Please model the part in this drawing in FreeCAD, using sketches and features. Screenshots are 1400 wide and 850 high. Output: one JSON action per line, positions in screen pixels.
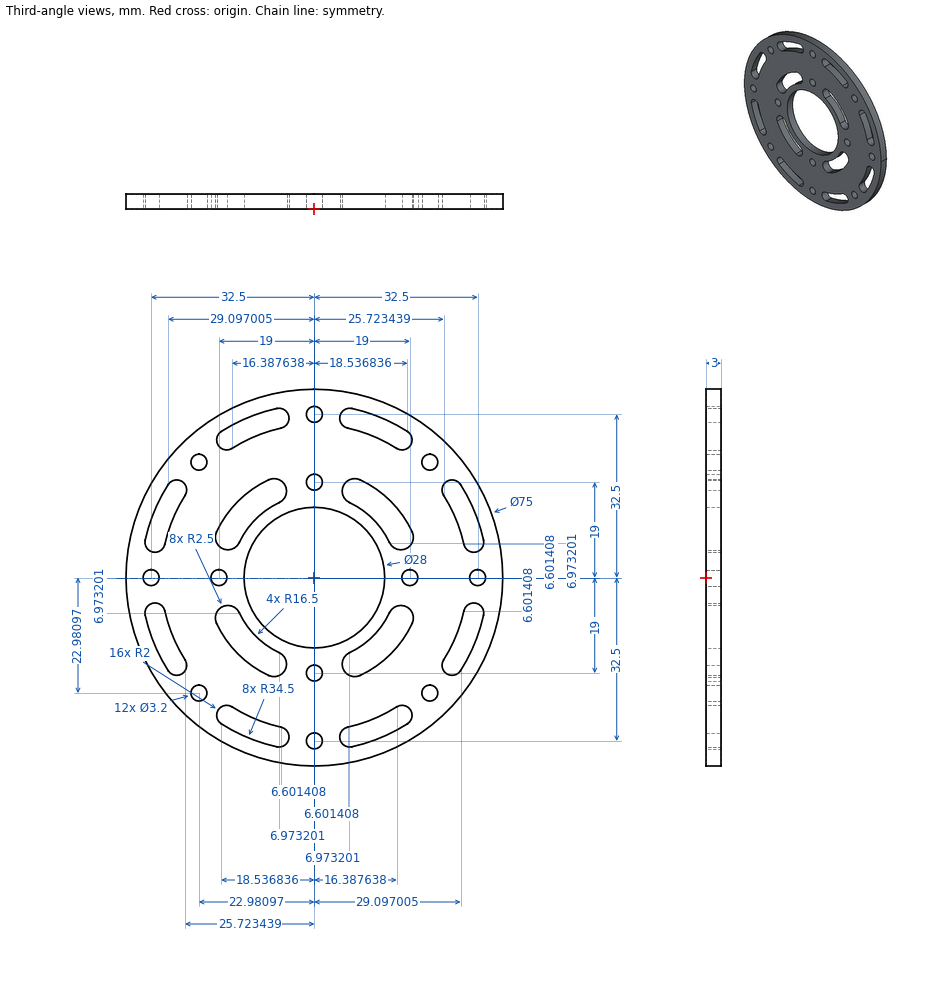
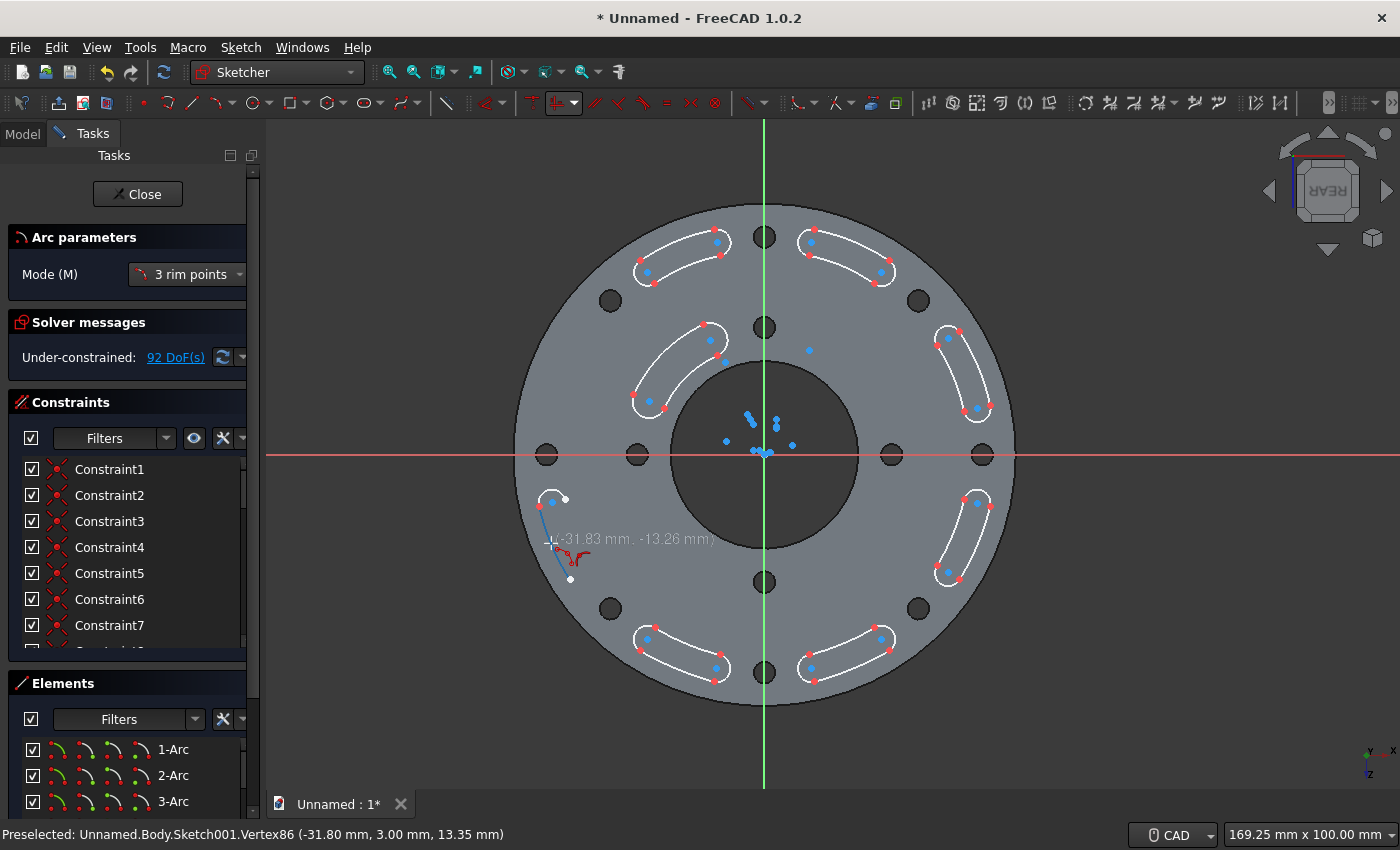
{"action": "left_click", "coordinate": [570, 580]}
{"action": "left_click", "coordinate": [592, 565]}
{"action": "left_click", "coordinate": [588, 583]}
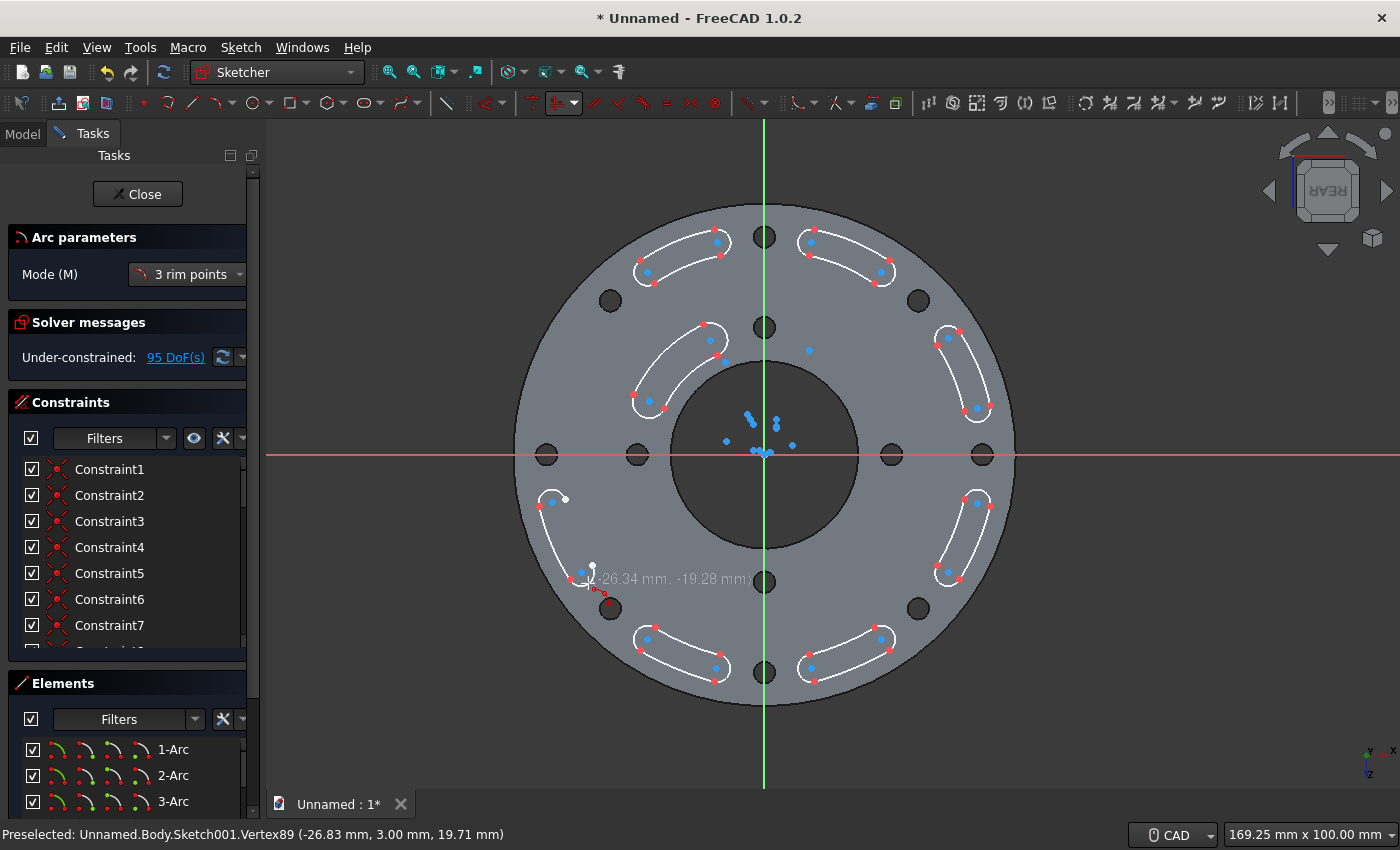
{"action": "left_click", "coordinate": [592, 566]}
{"action": "left_click", "coordinate": [565, 500]}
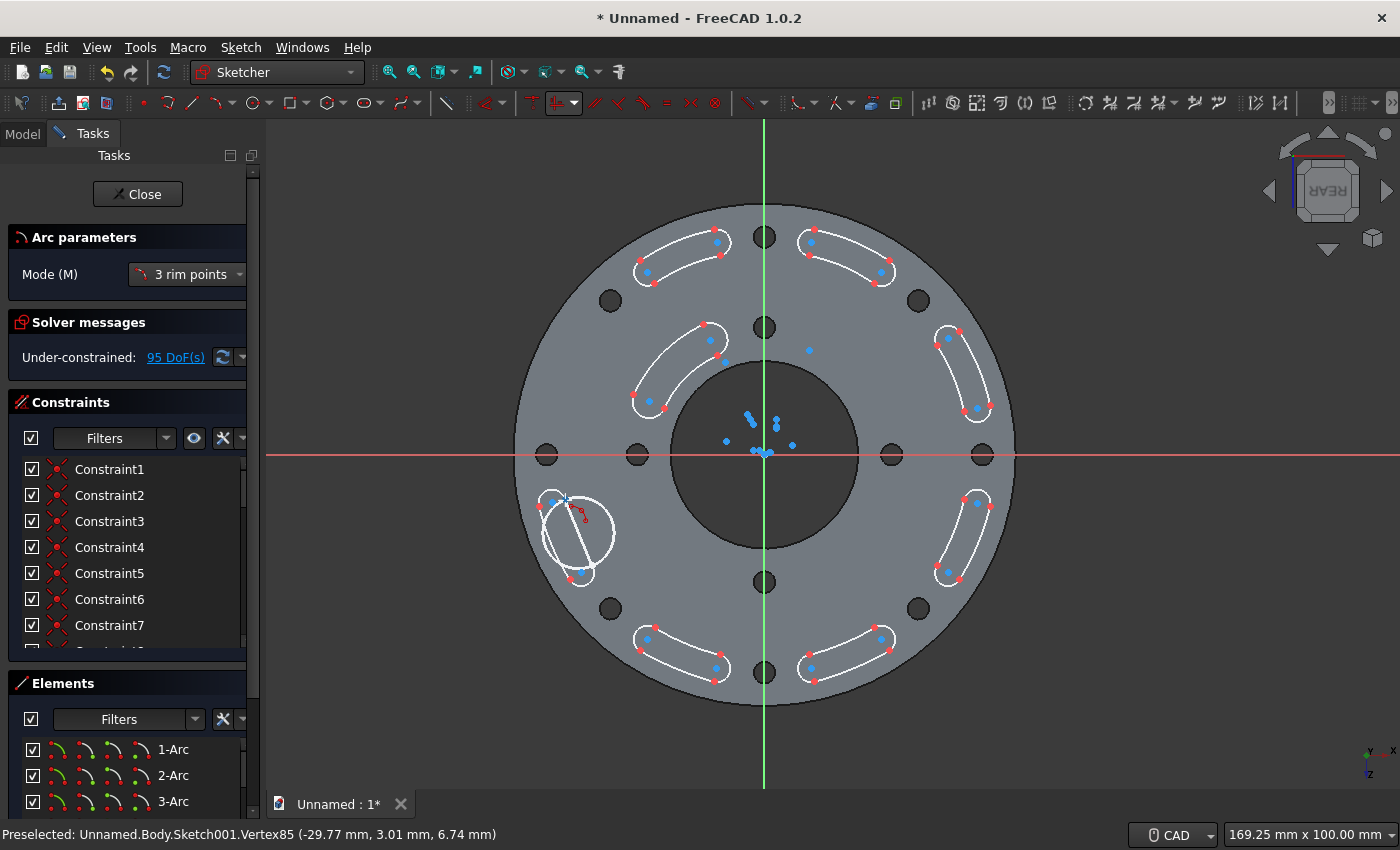
{"action": "scroll", "coordinate": [576, 533], "scroll_direction": "up", "scroll_amount": 9}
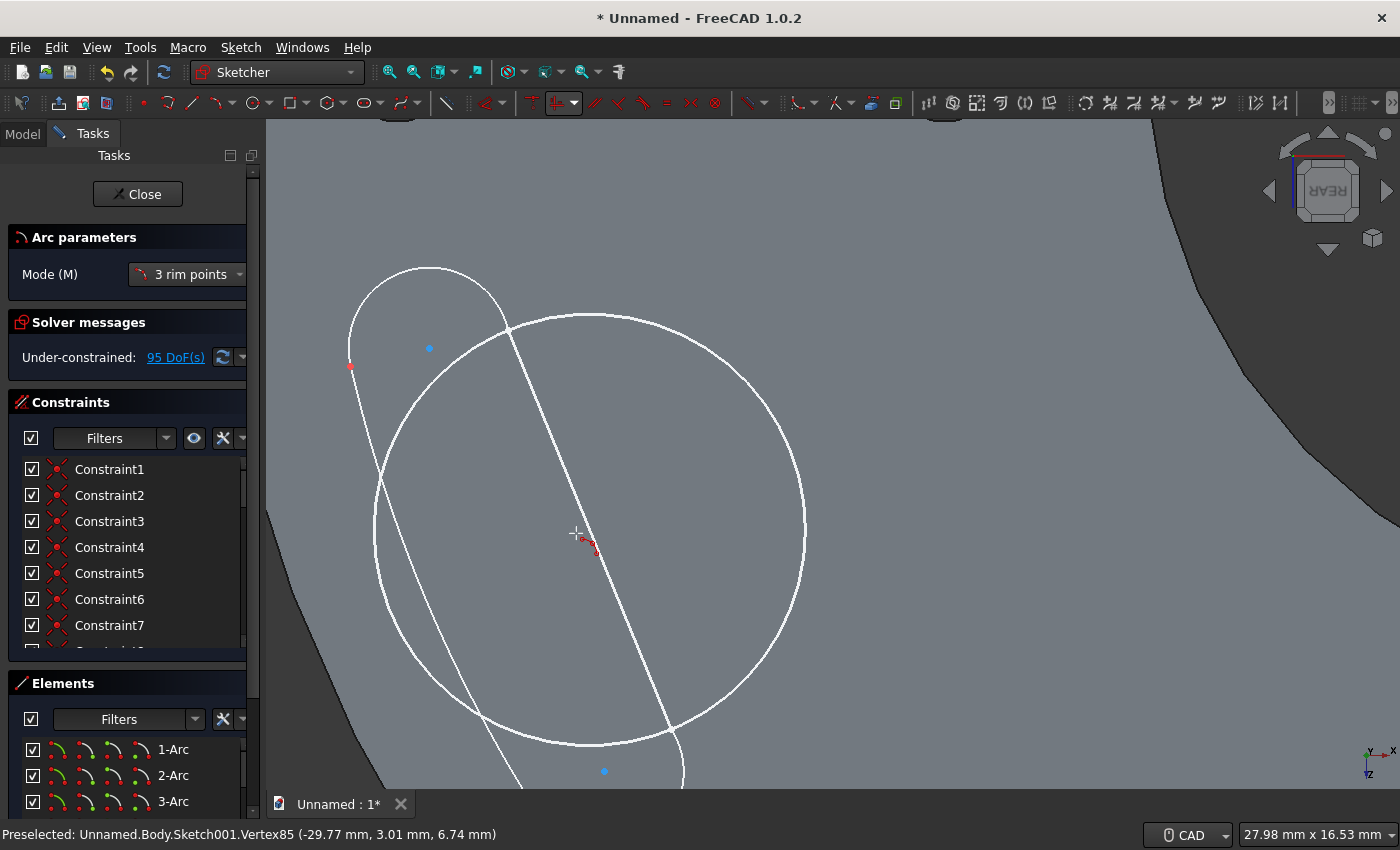
{"action": "left_click", "coordinate": [573, 530]}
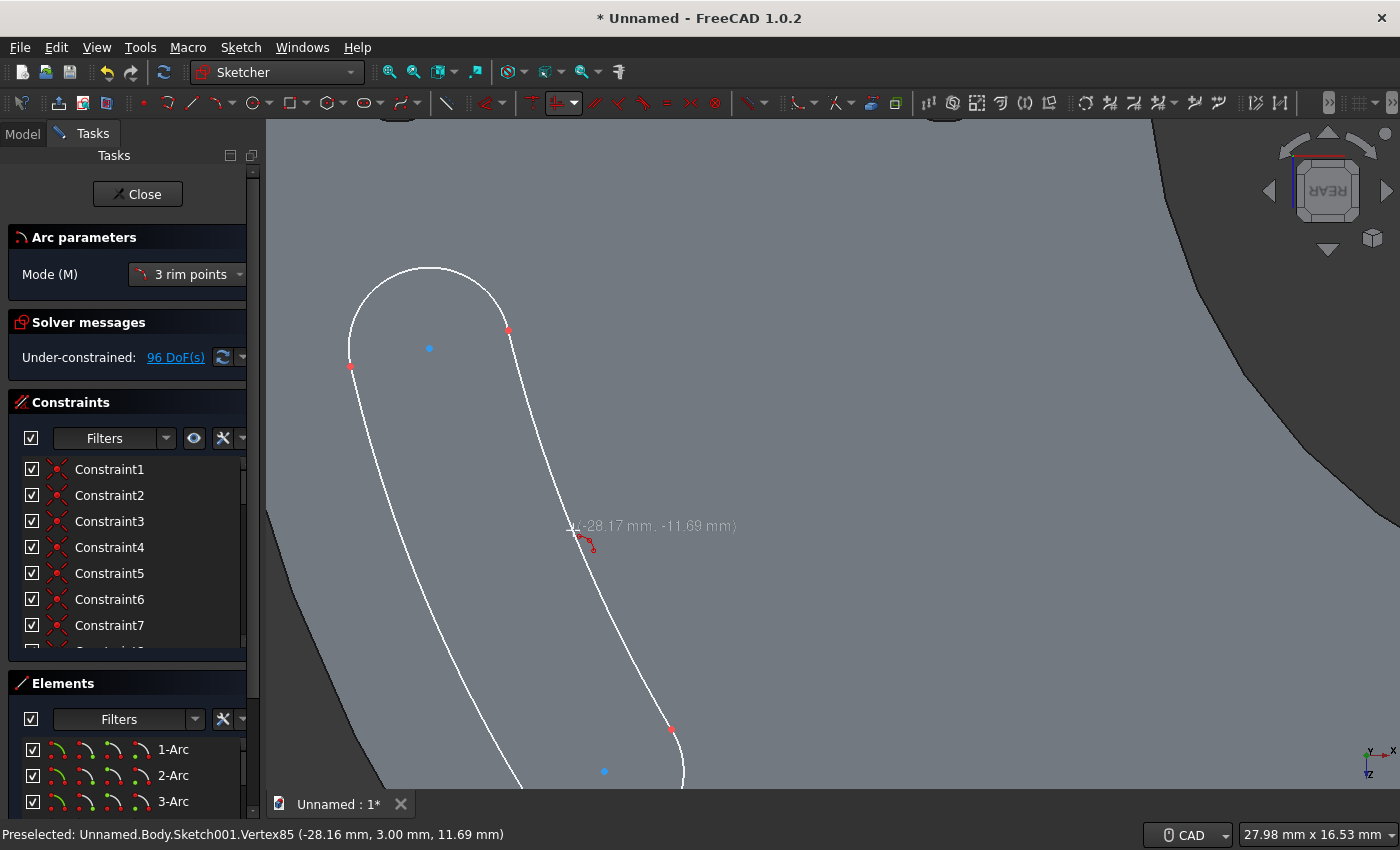
{"action": "scroll", "coordinate": [576, 533], "scroll_direction": "down", "scroll_amount": 9}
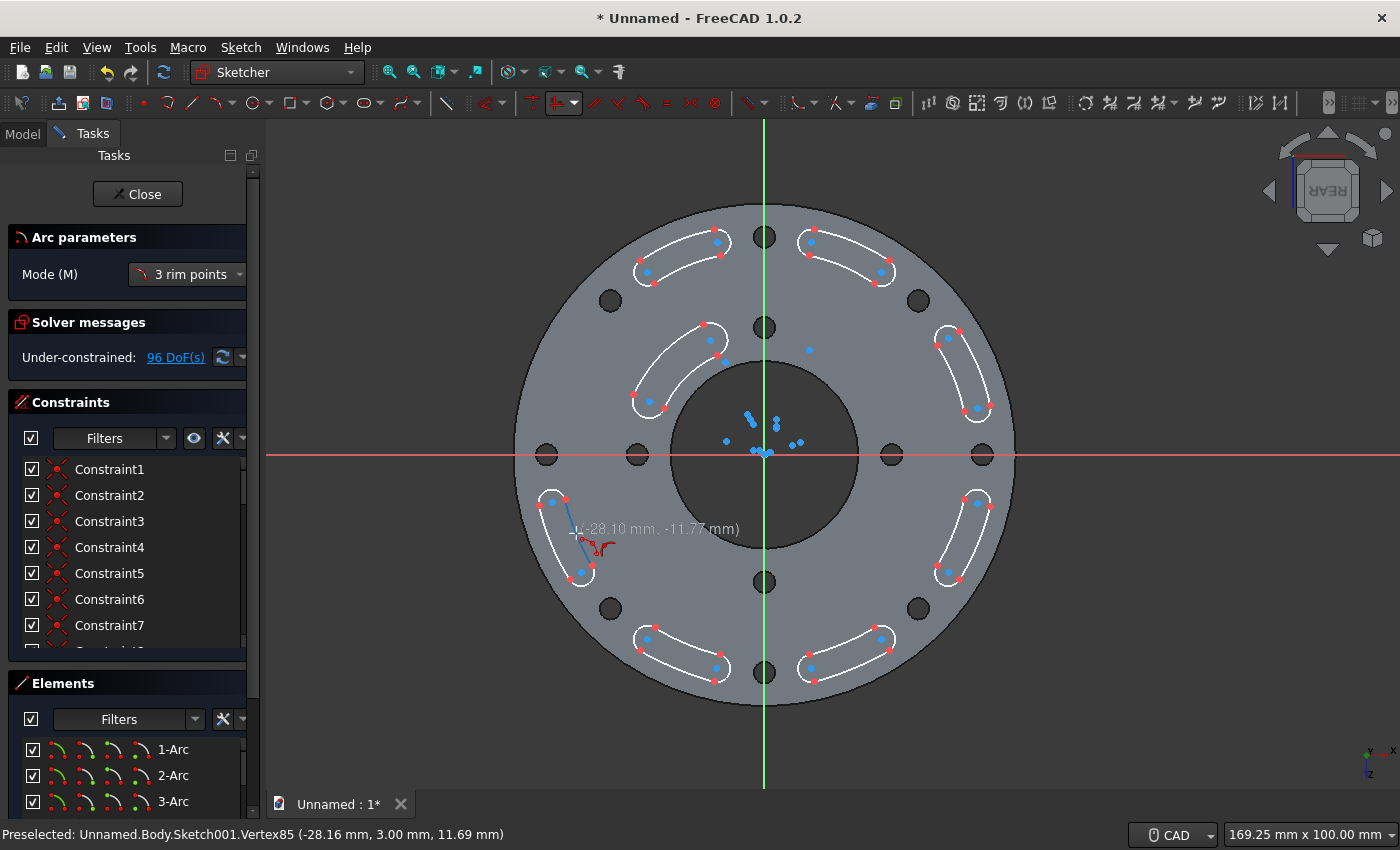
{"action": "left_click", "coordinate": [565, 411]}
{"action": "left_click", "coordinate": [592, 345]}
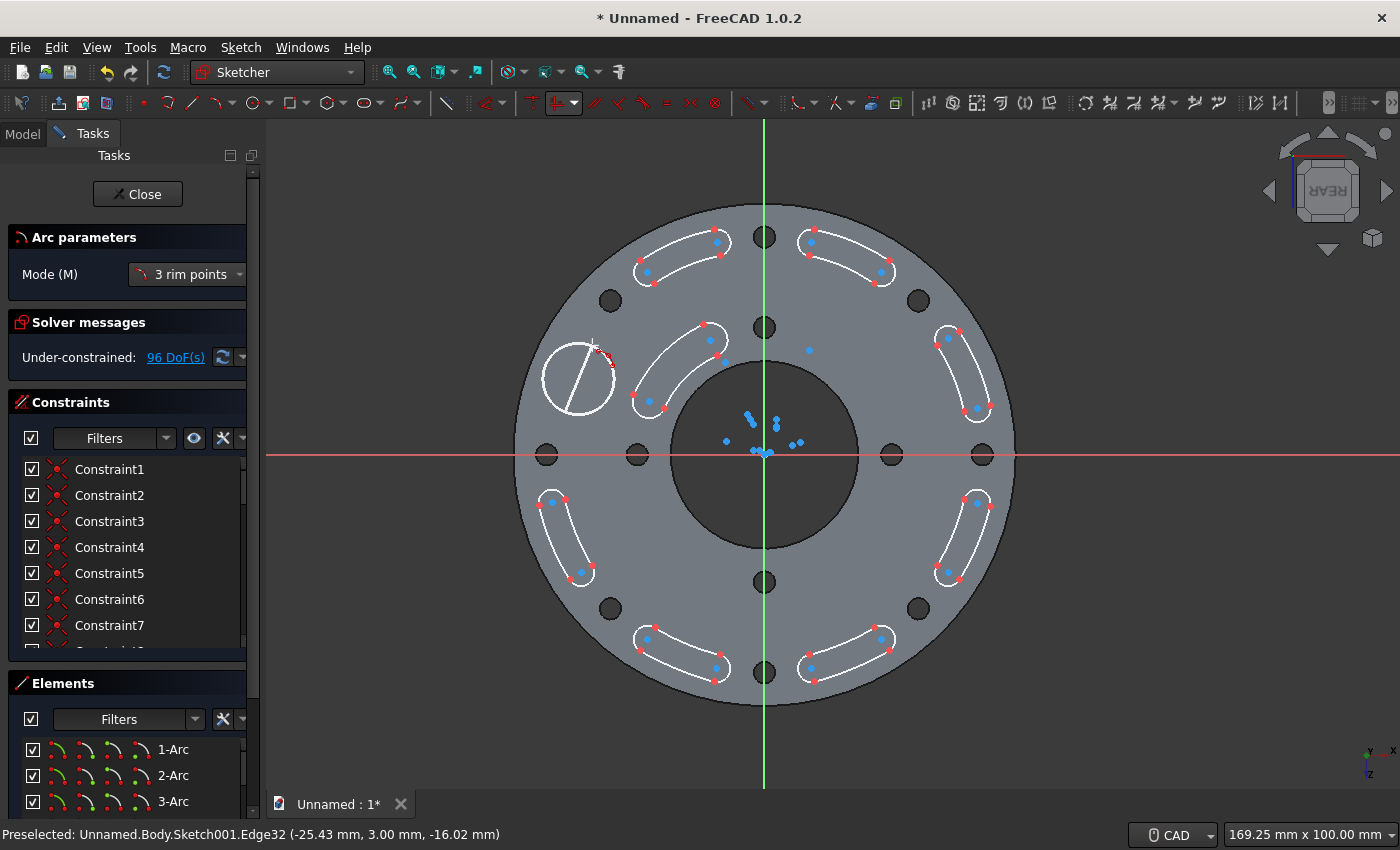
{"action": "scroll", "coordinate": [576, 377], "scroll_direction": "up", "scroll_amount": 9}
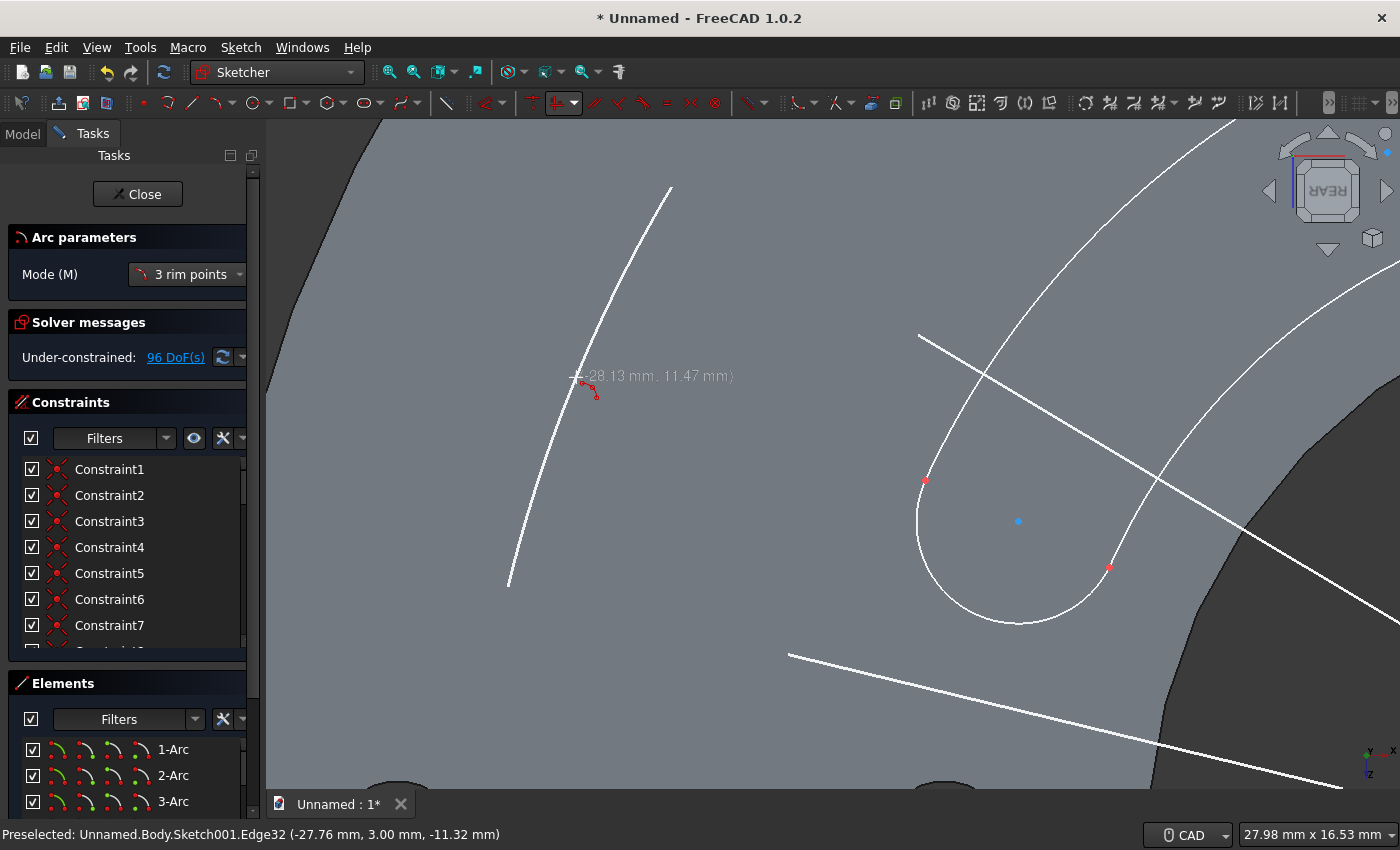
{"action": "left_click", "coordinate": [573, 373]}